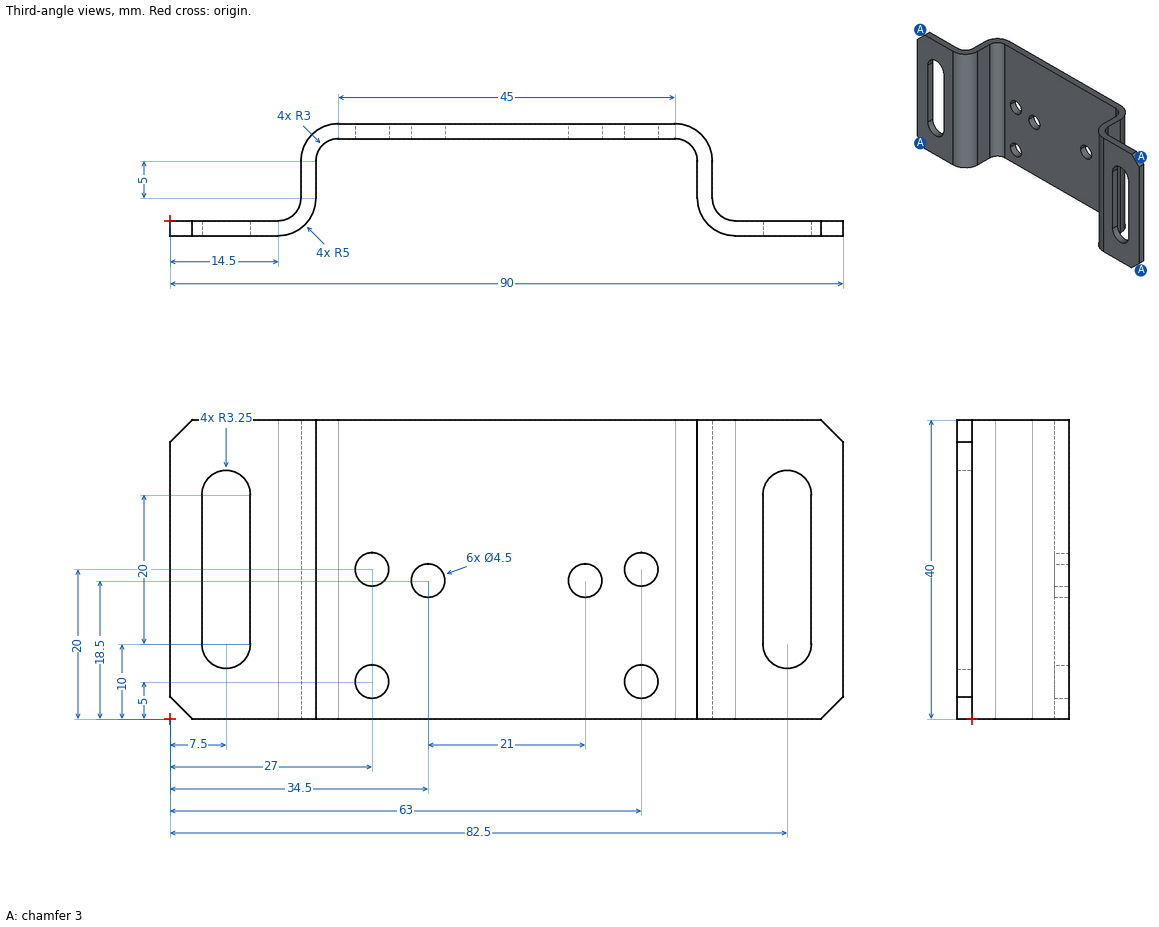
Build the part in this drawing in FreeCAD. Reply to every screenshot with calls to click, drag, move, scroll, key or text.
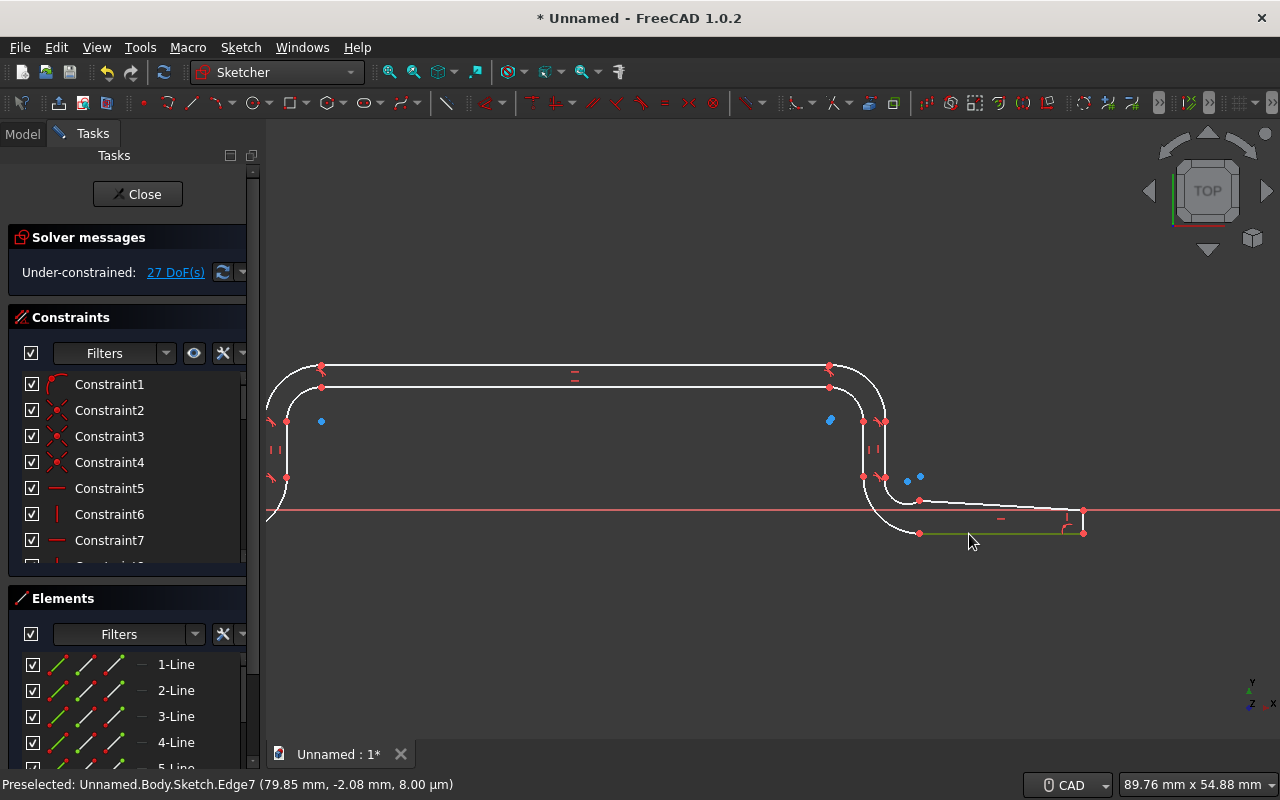
click(894, 527)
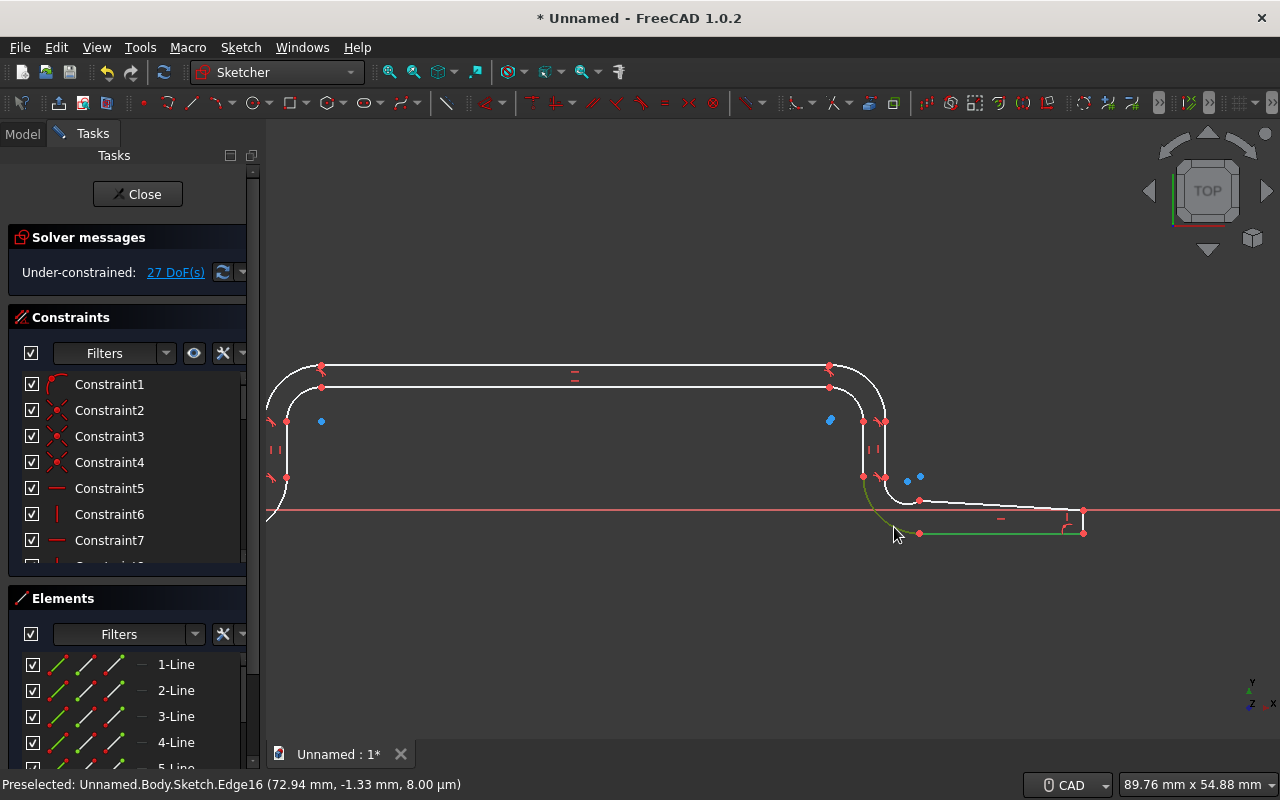
key(t)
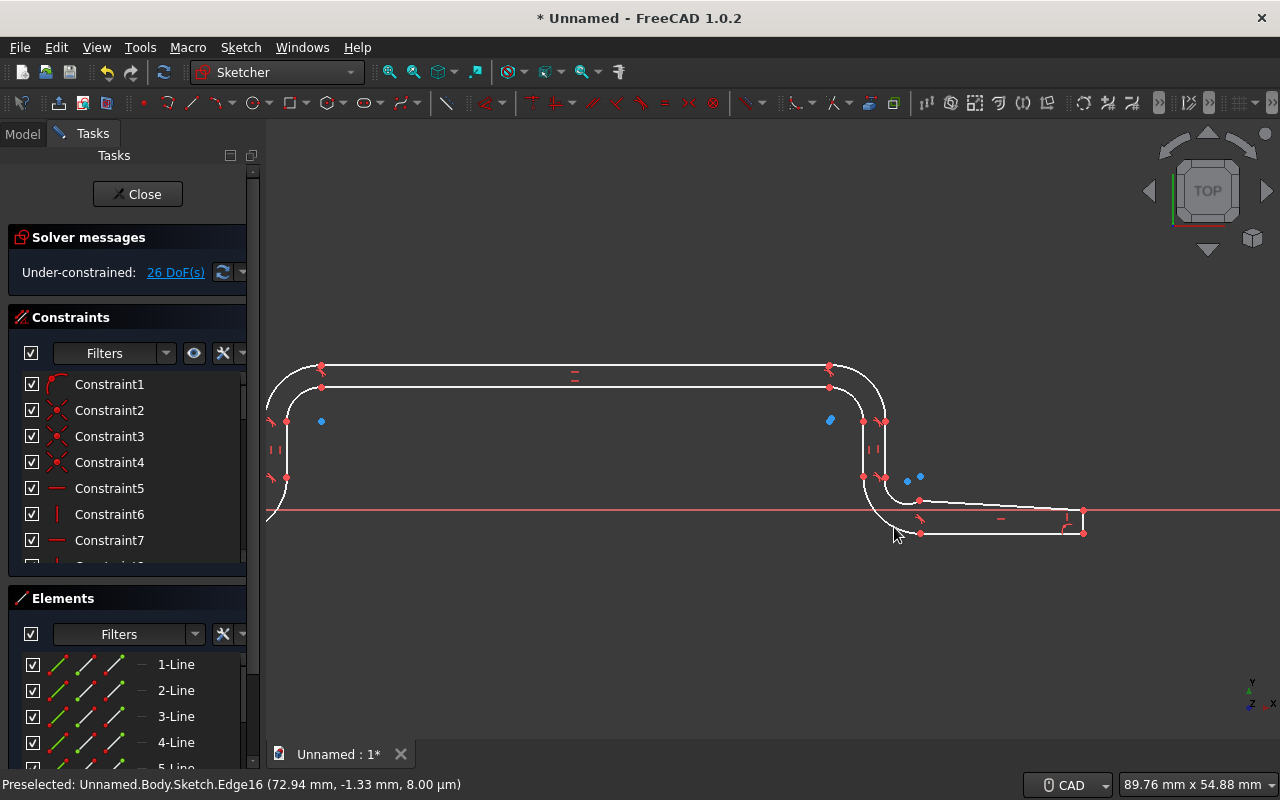
click(1034, 507)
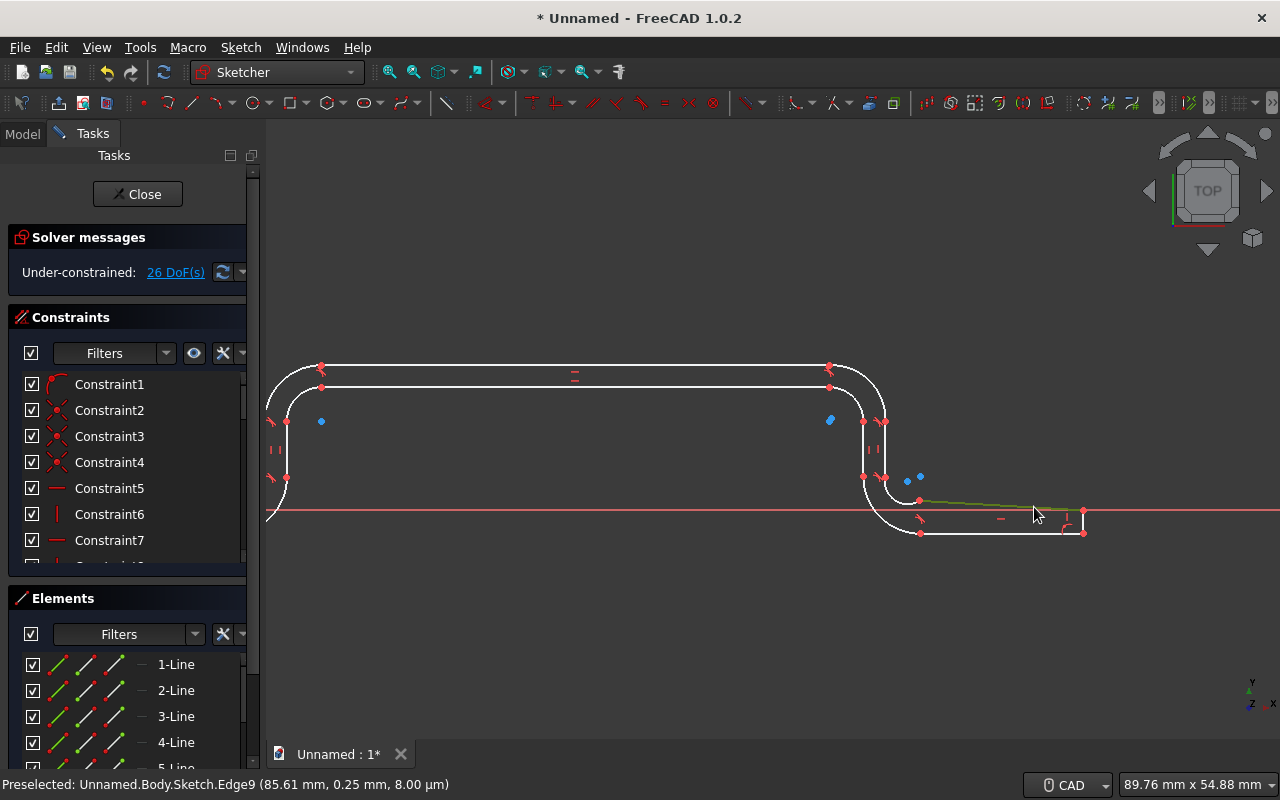
click(888, 493)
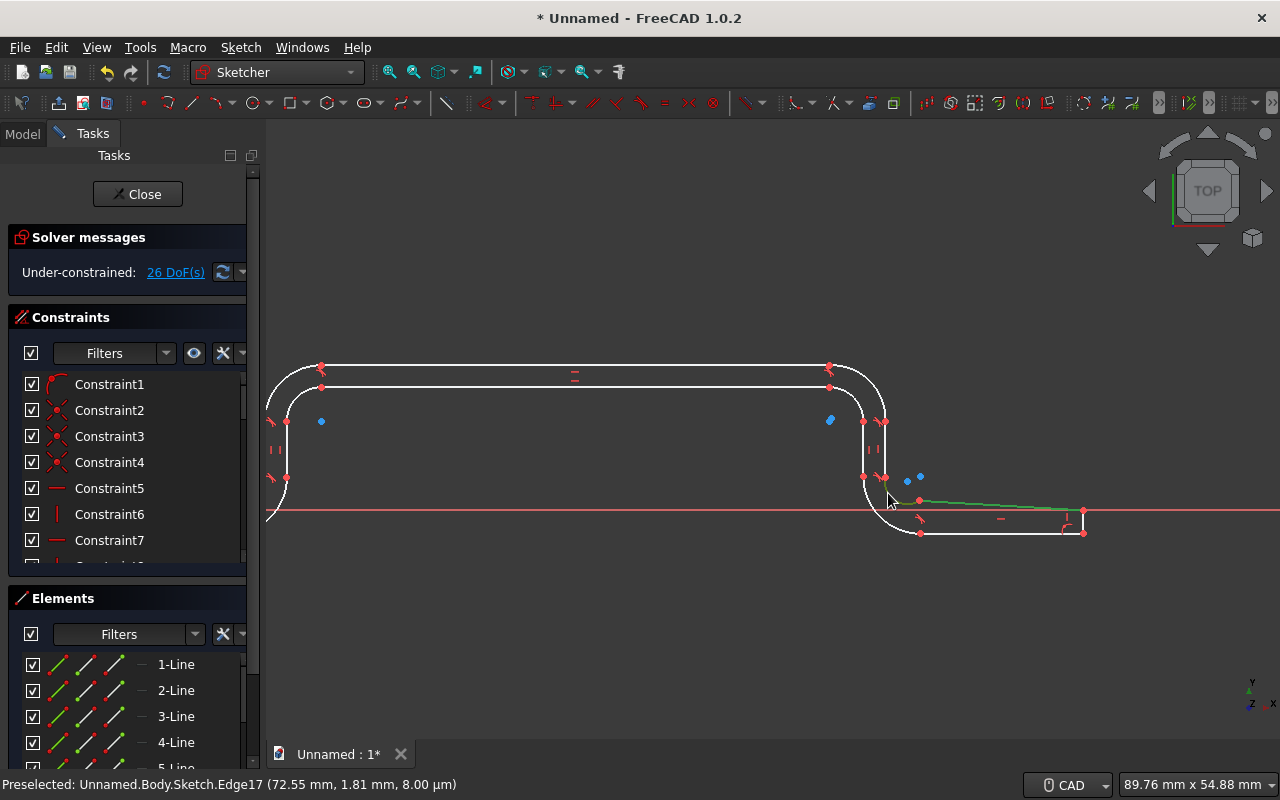
key(t)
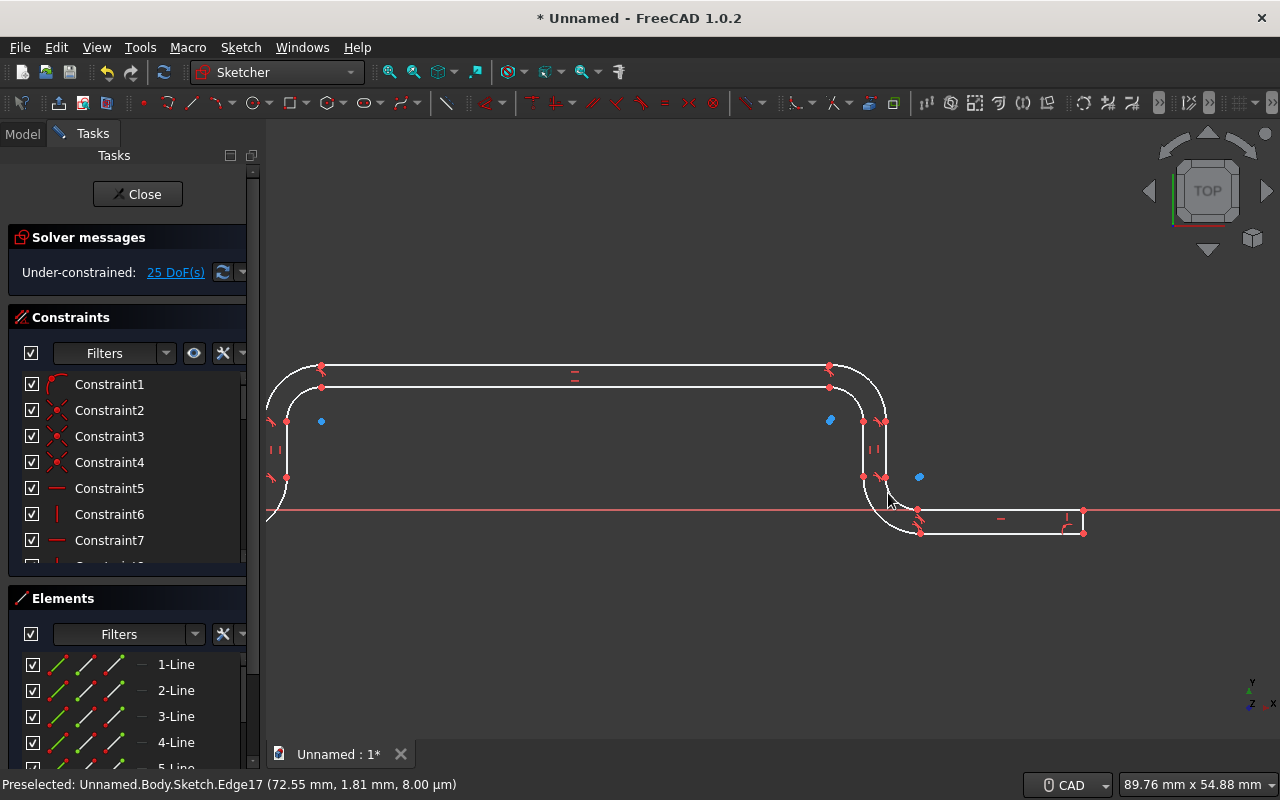
click(886, 461)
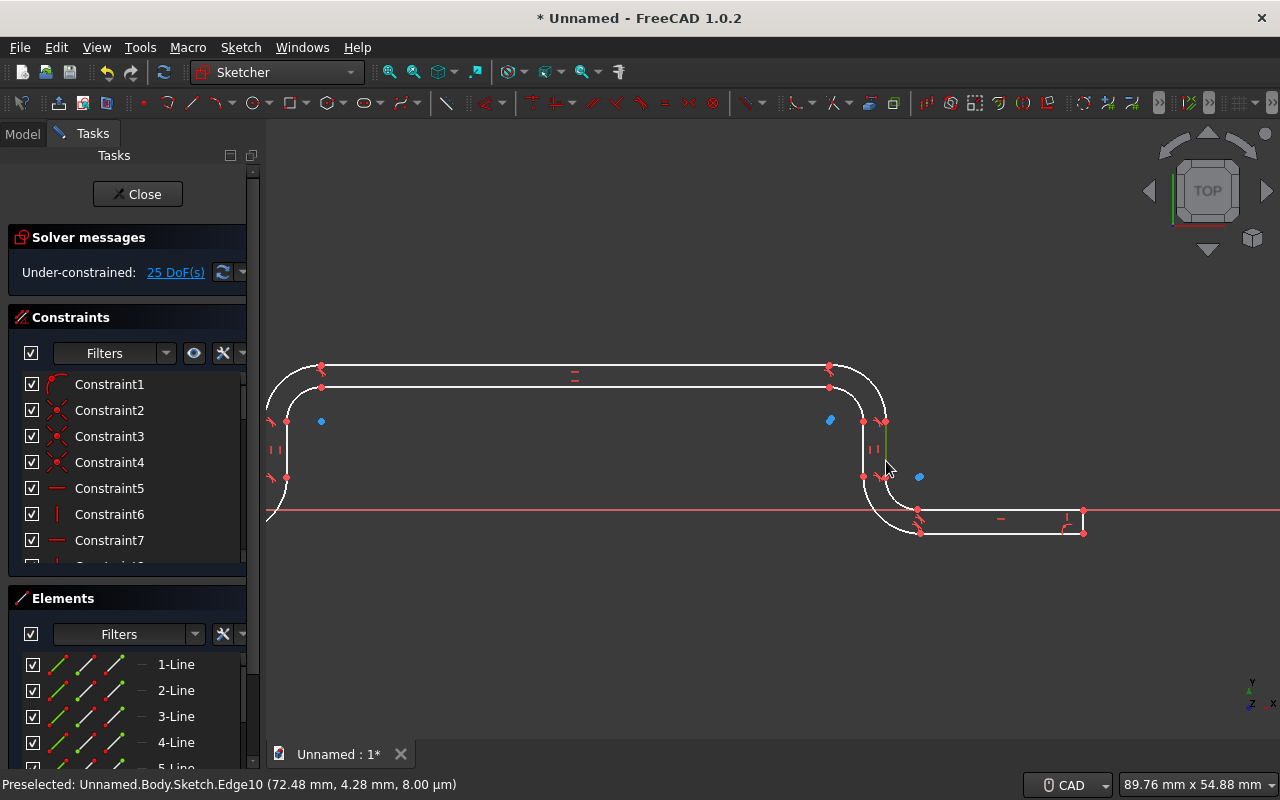
click(889, 492)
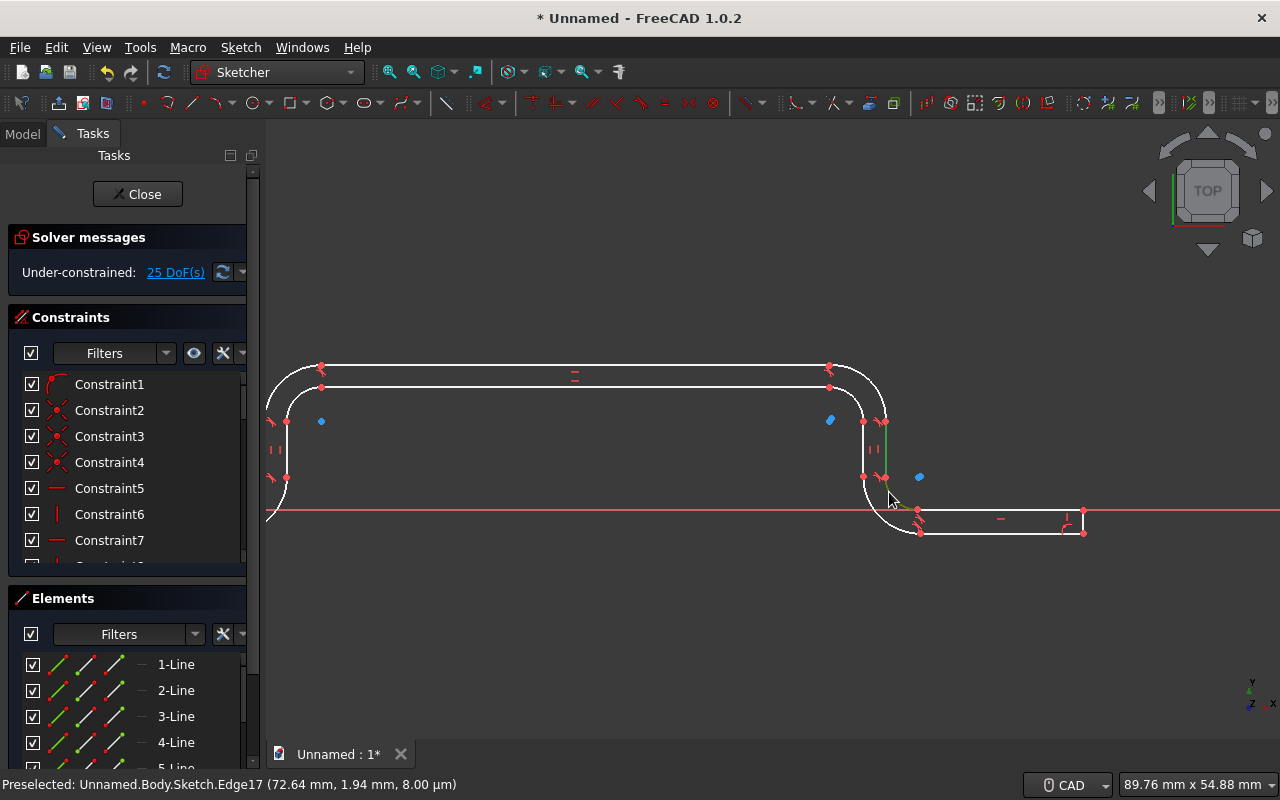
click(642, 104)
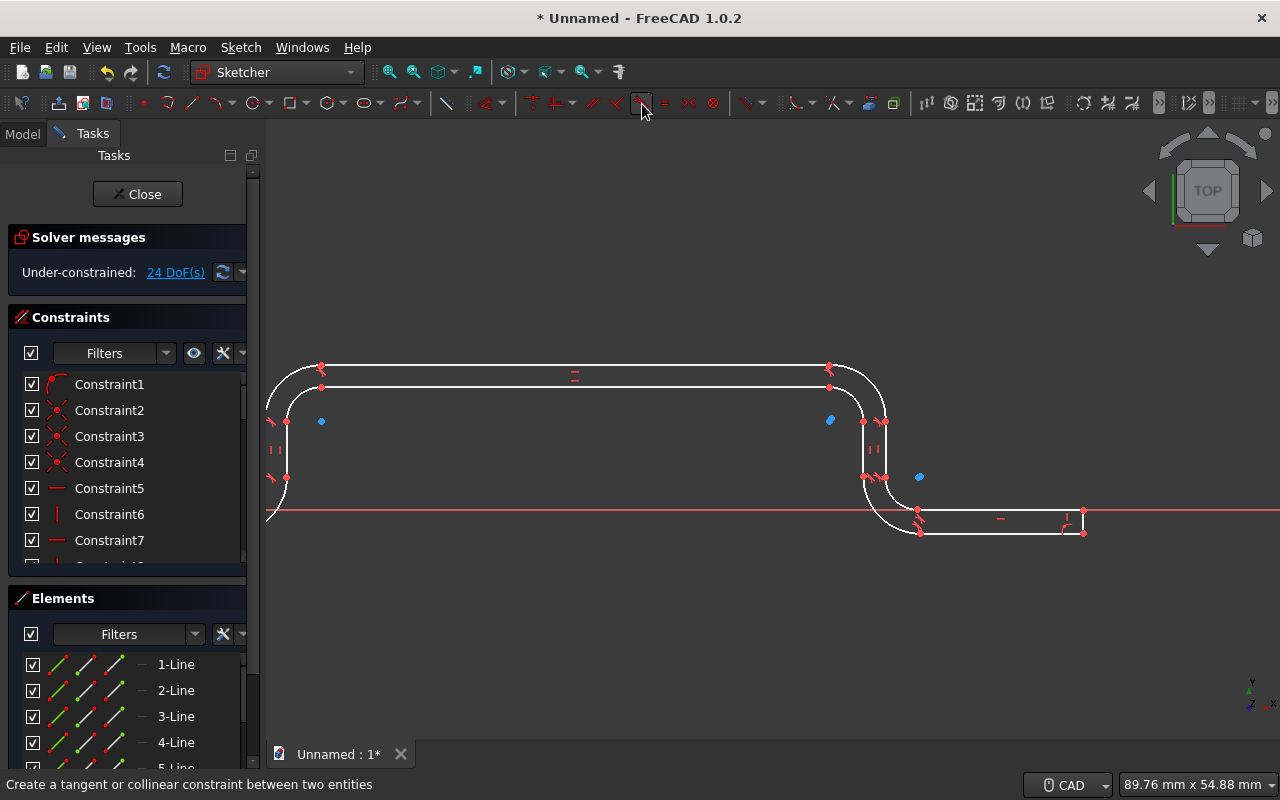
click(886, 461)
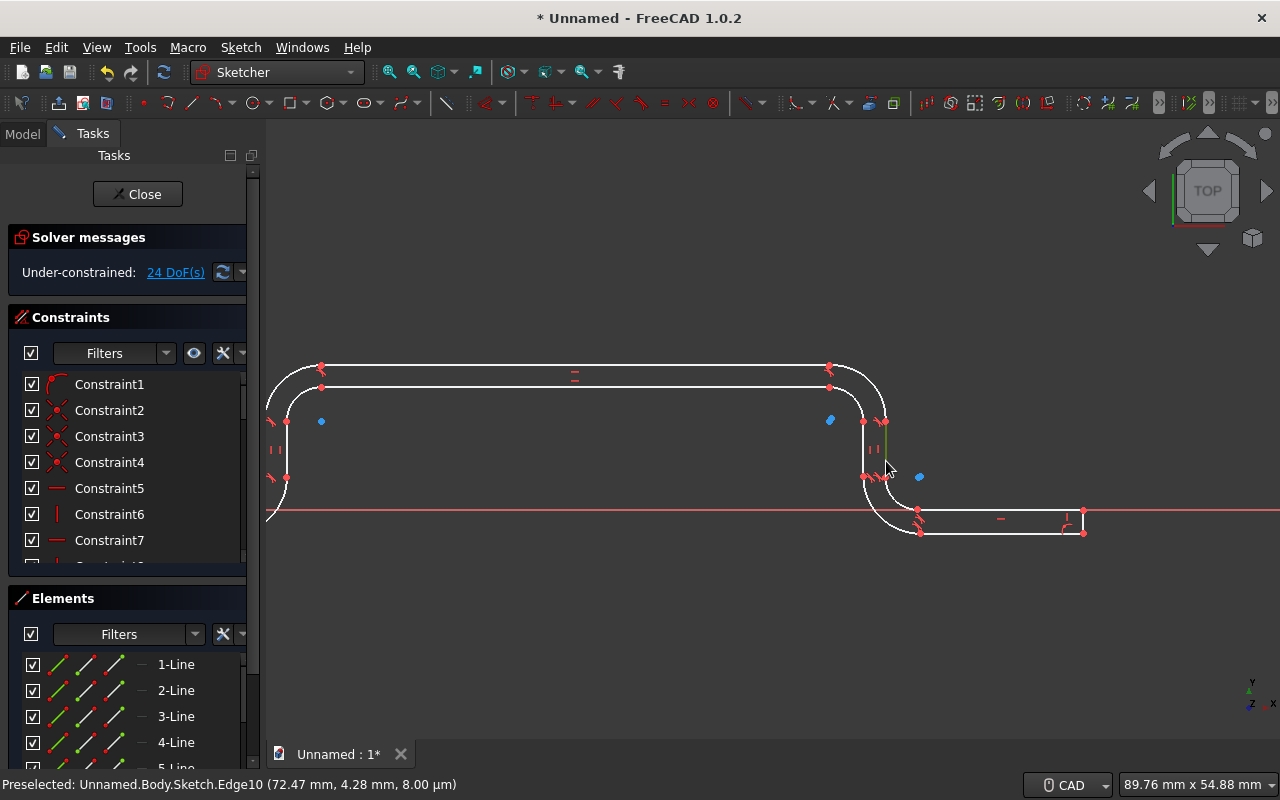
click(880, 395)